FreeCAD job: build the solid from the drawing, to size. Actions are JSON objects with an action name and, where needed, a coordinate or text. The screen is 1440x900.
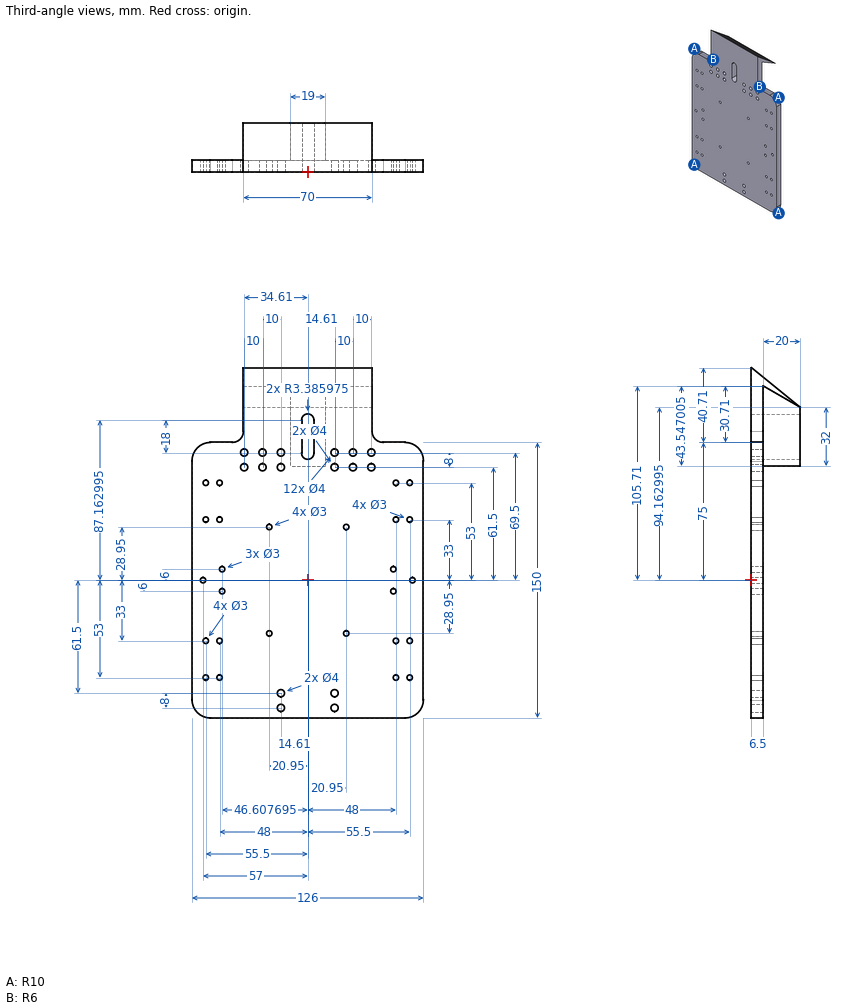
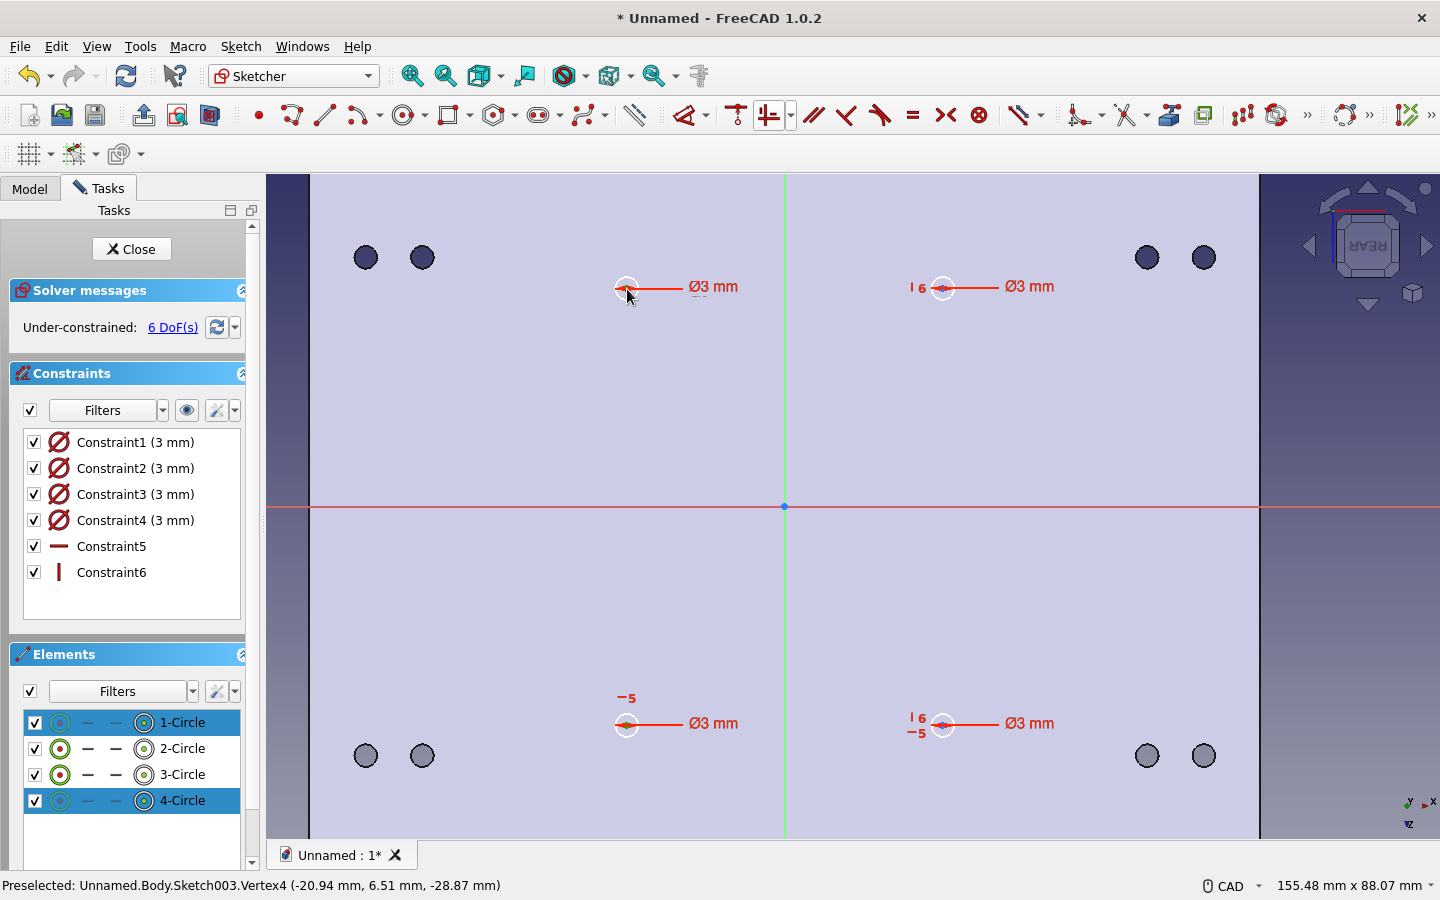
{"action": "left_click", "coordinate": [790, 116]}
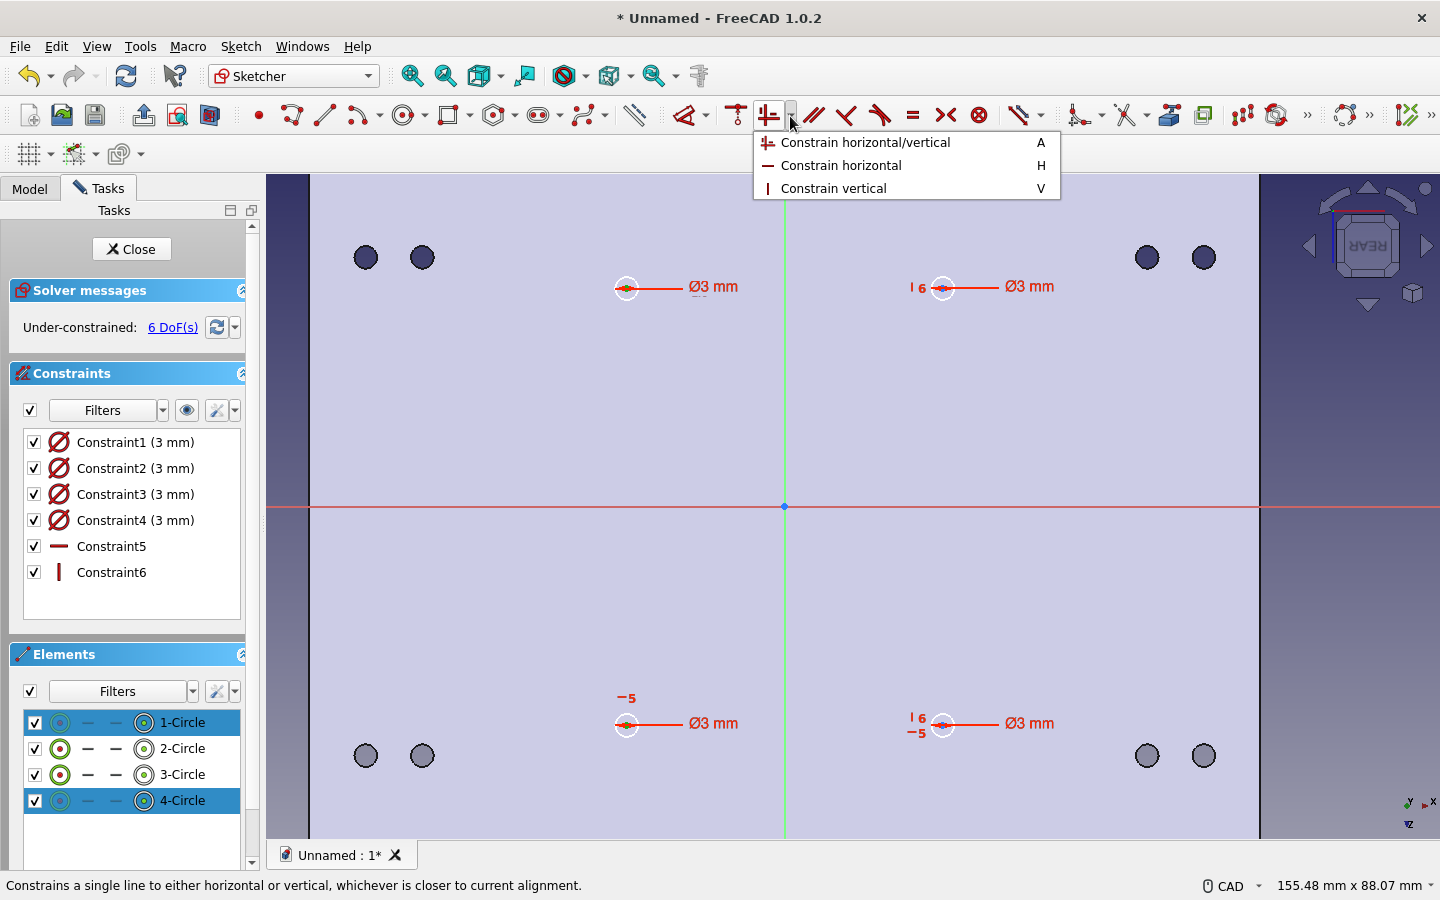
{"action": "left_click", "coordinate": [907, 188]}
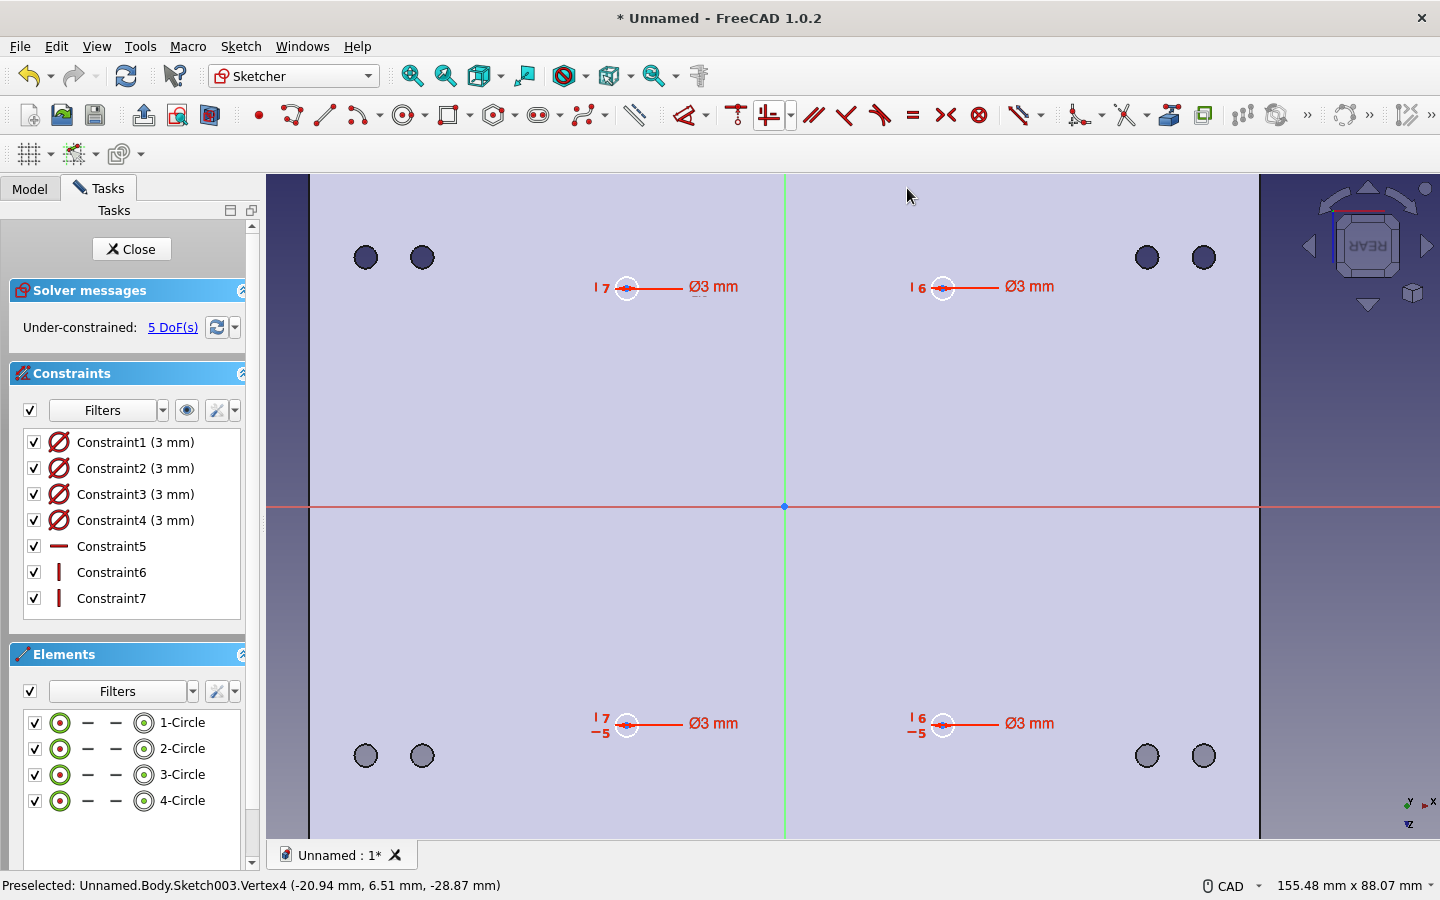
{"action": "left_click", "coordinate": [943, 288]}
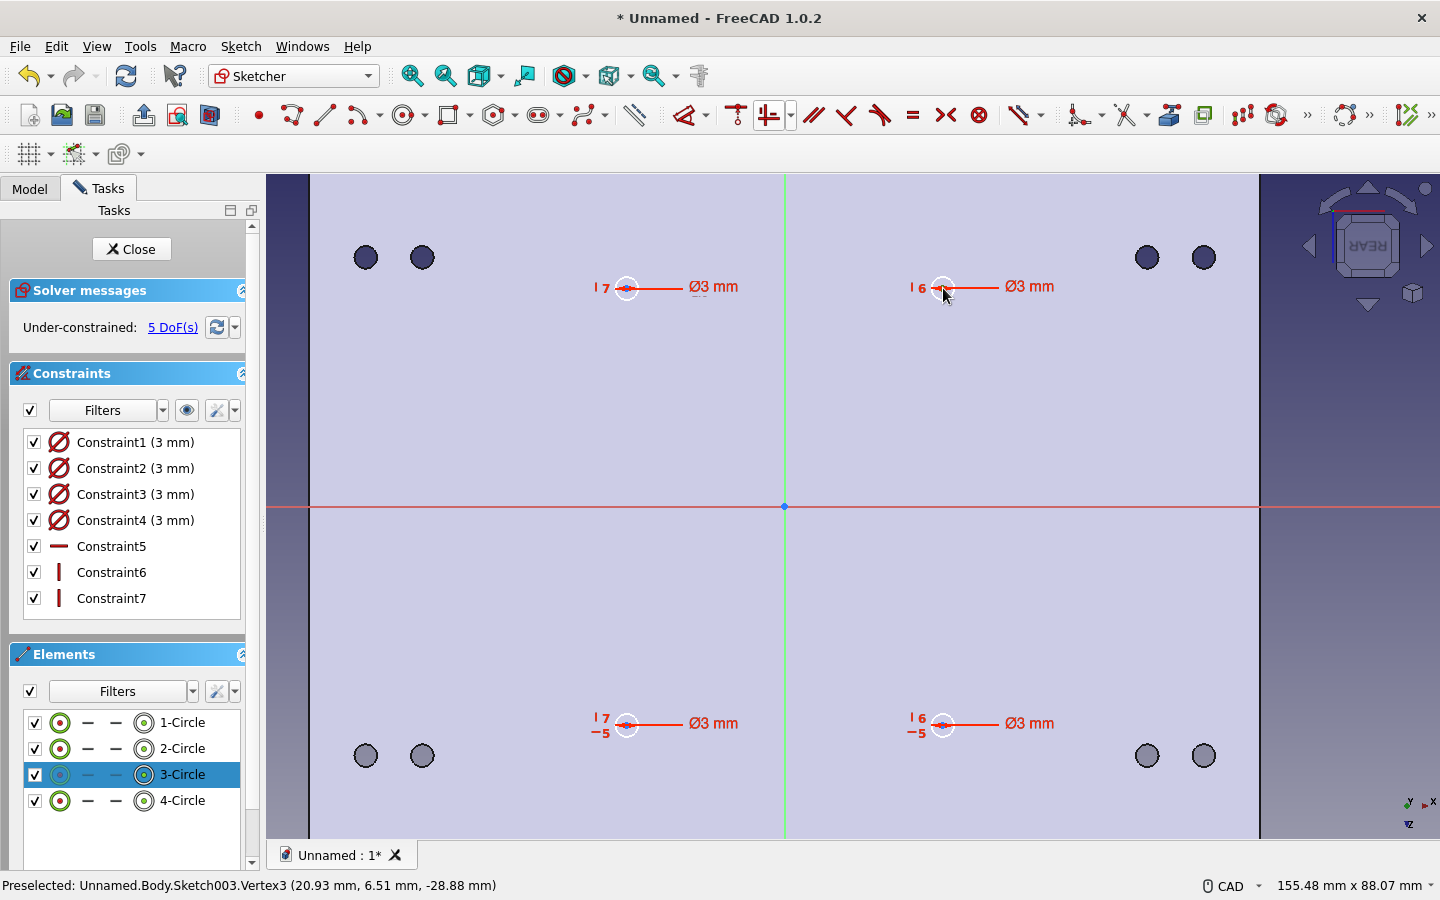
{"action": "left_click", "coordinate": [627, 289]}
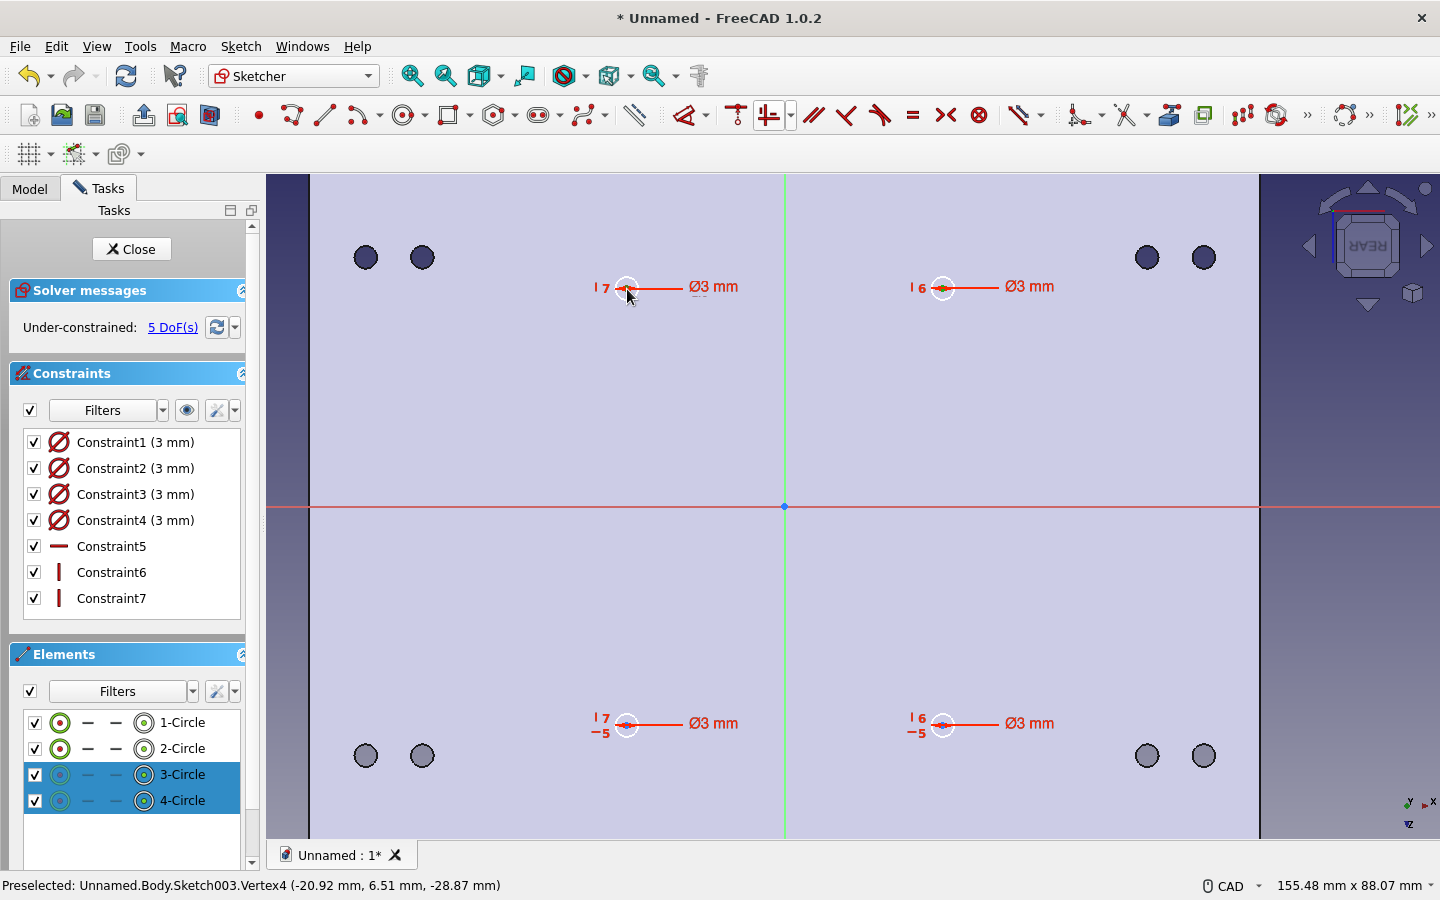
{"action": "left_click", "coordinate": [790, 116]}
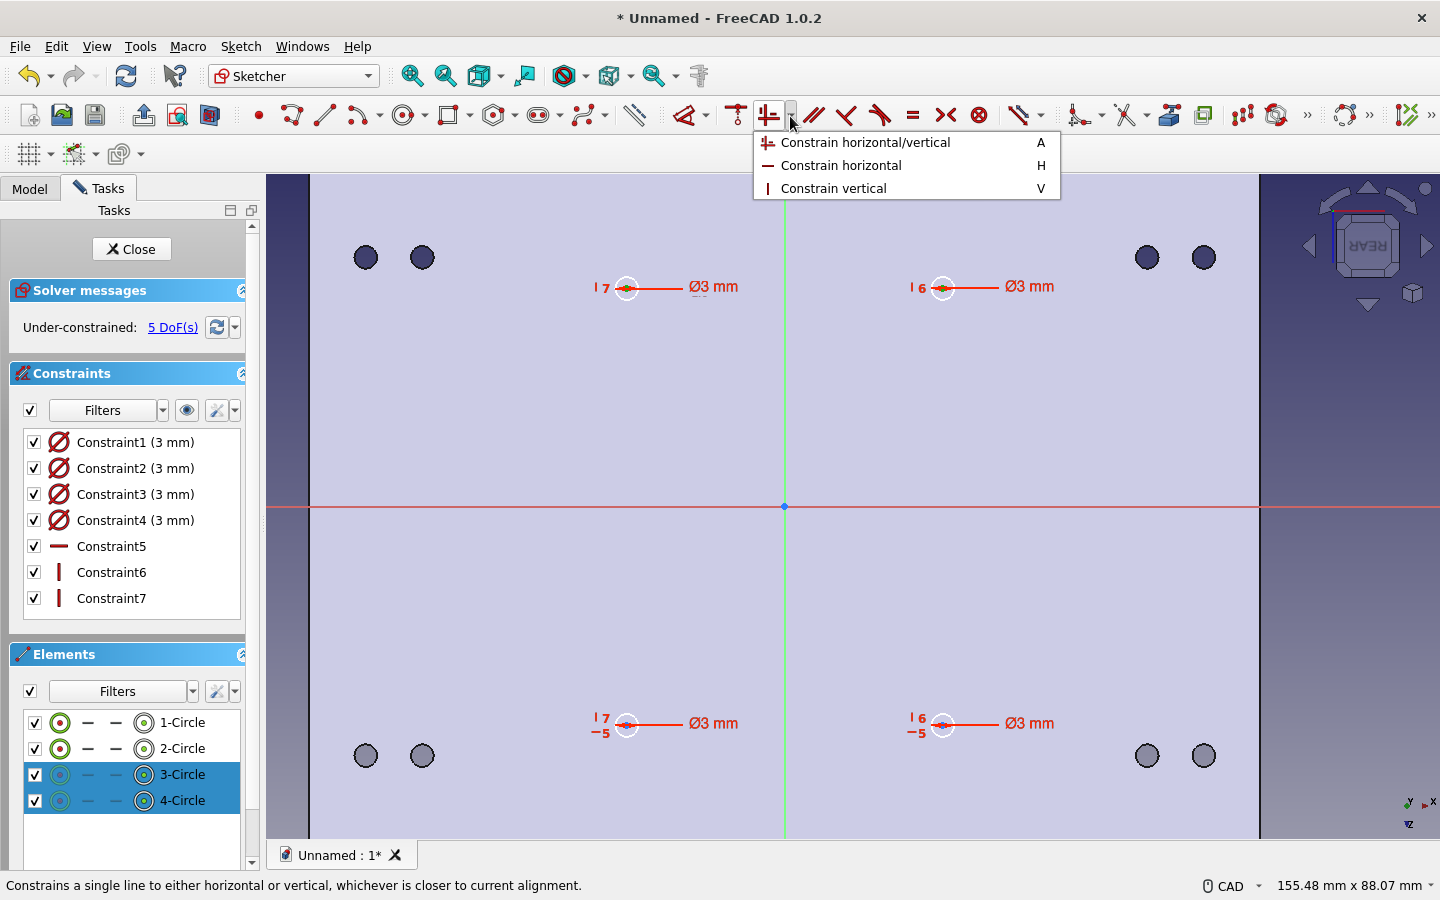
{"action": "left_click", "coordinate": [907, 166]}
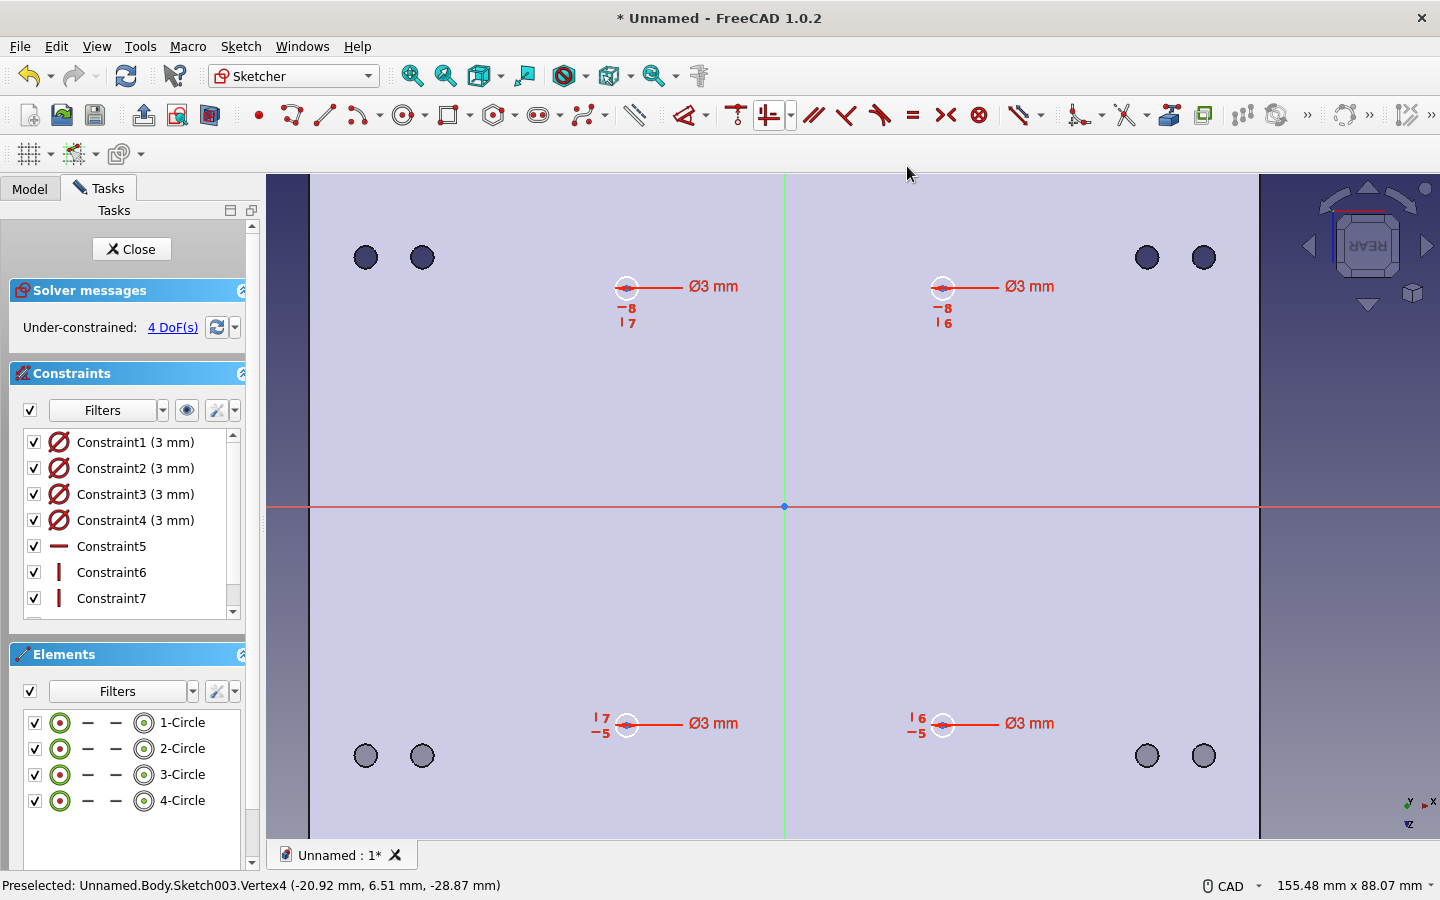
{"action": "left_click", "coordinate": [684, 116]}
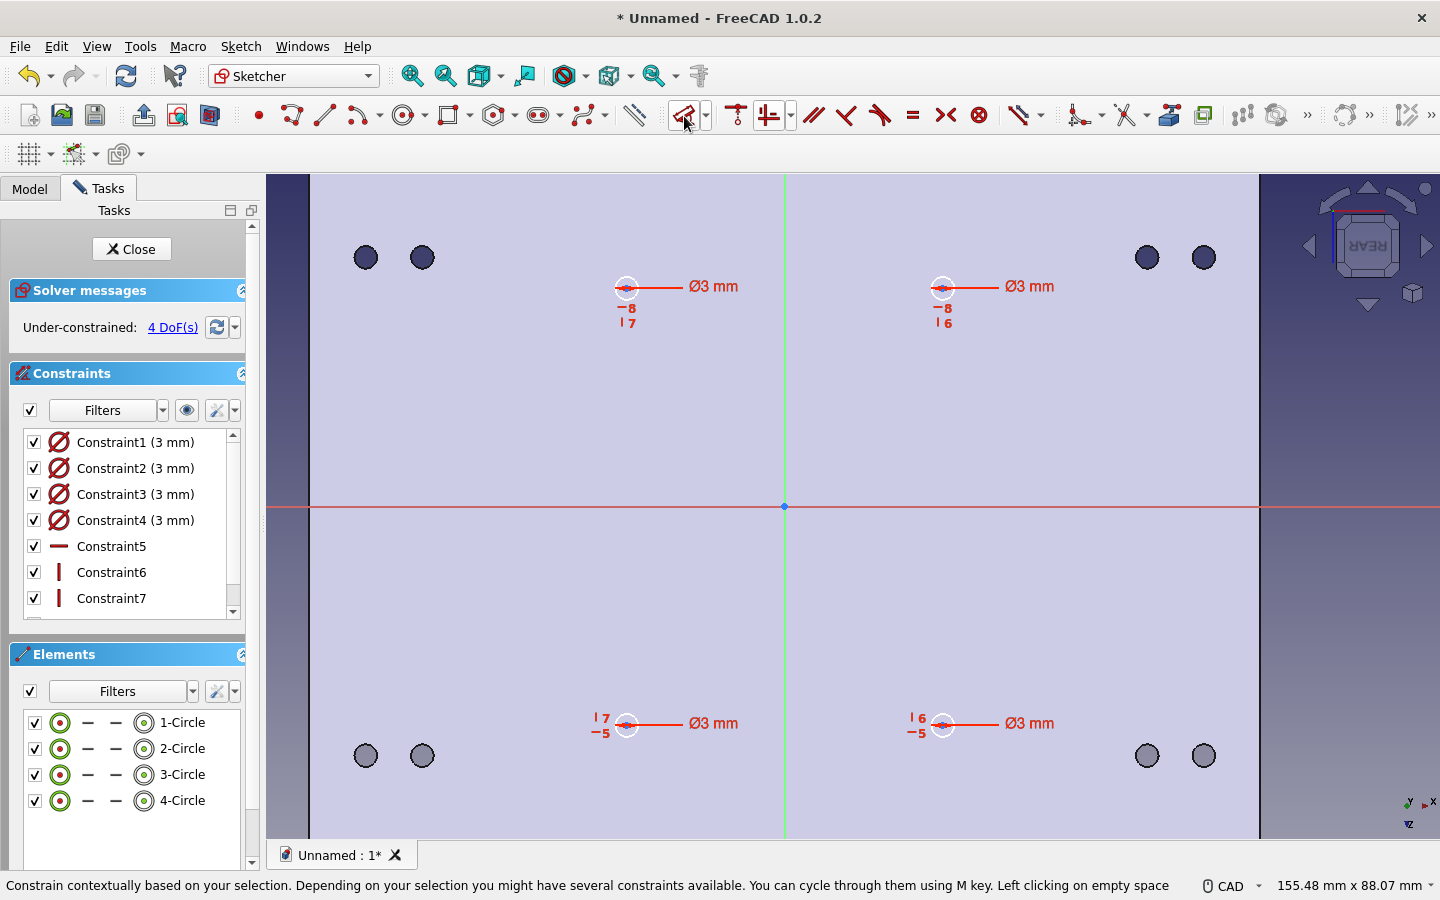
{"action": "left_click", "coordinate": [627, 725]}
{"action": "left_click", "coordinate": [706, 759]}